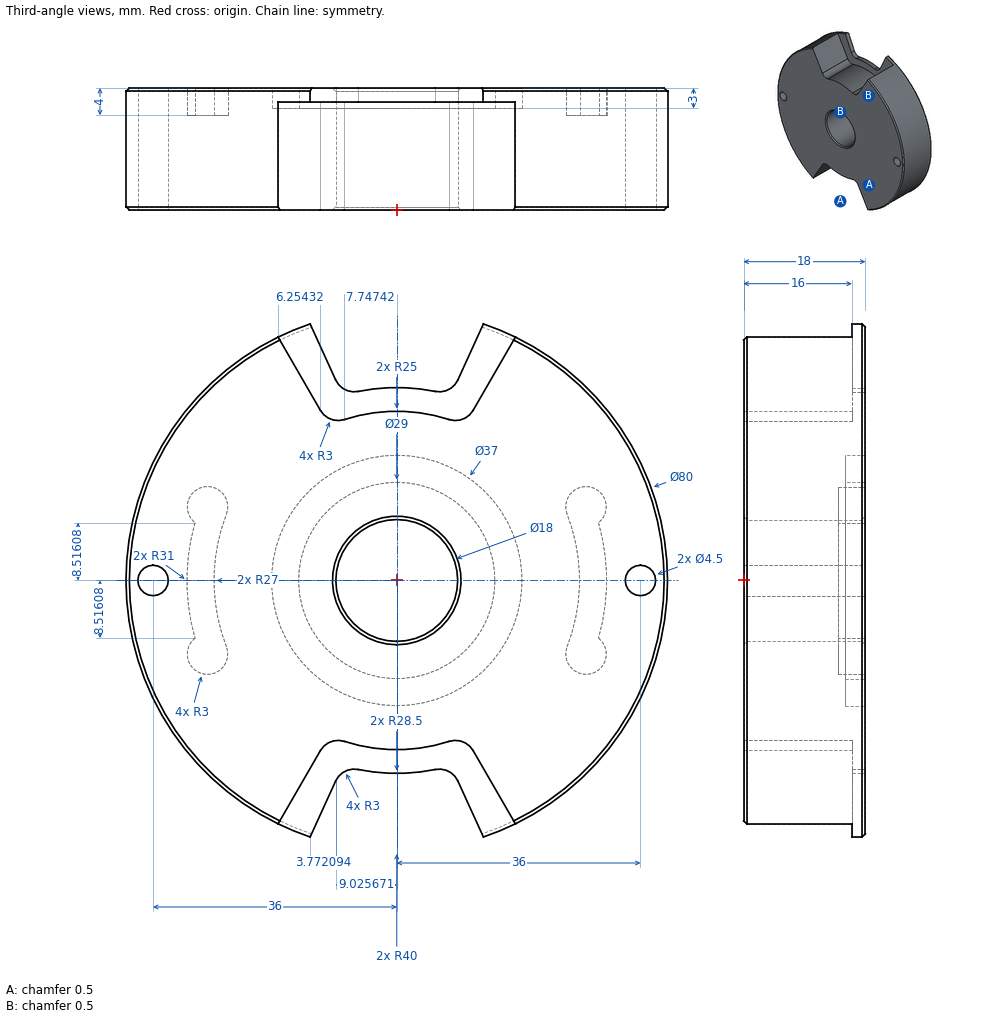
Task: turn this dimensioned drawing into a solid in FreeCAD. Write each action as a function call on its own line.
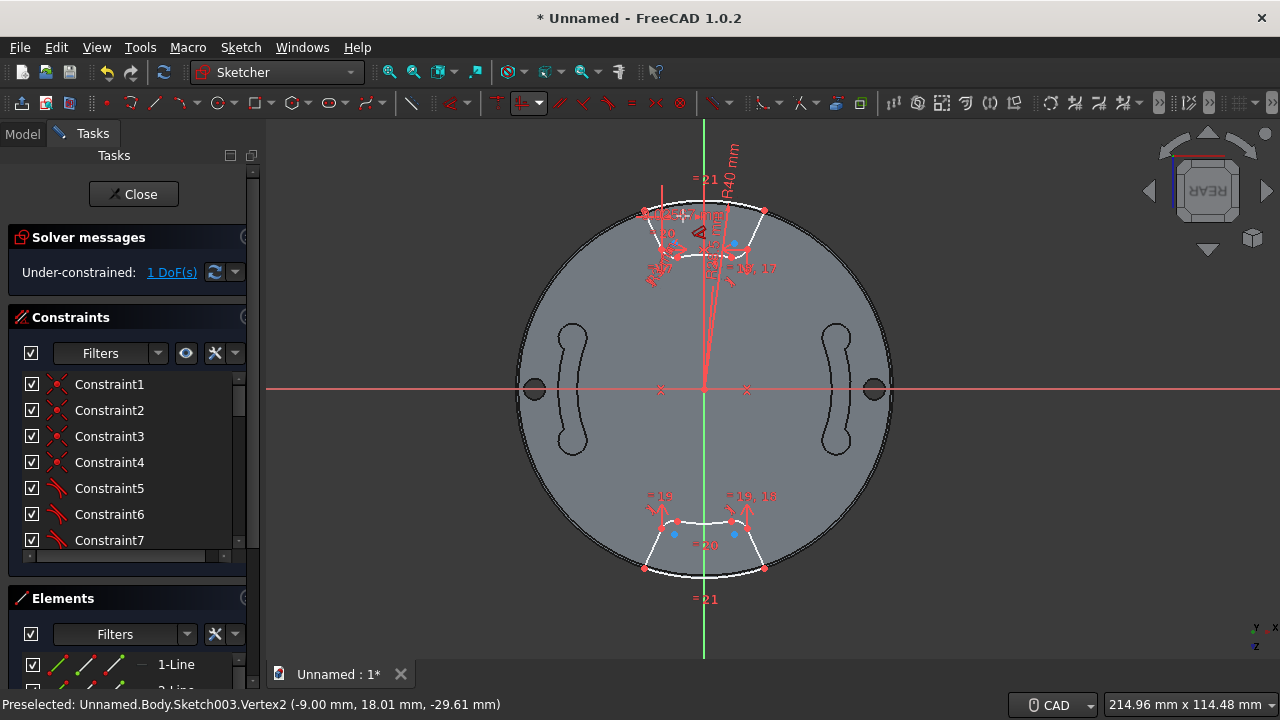
scroll(649, 222, up, 5)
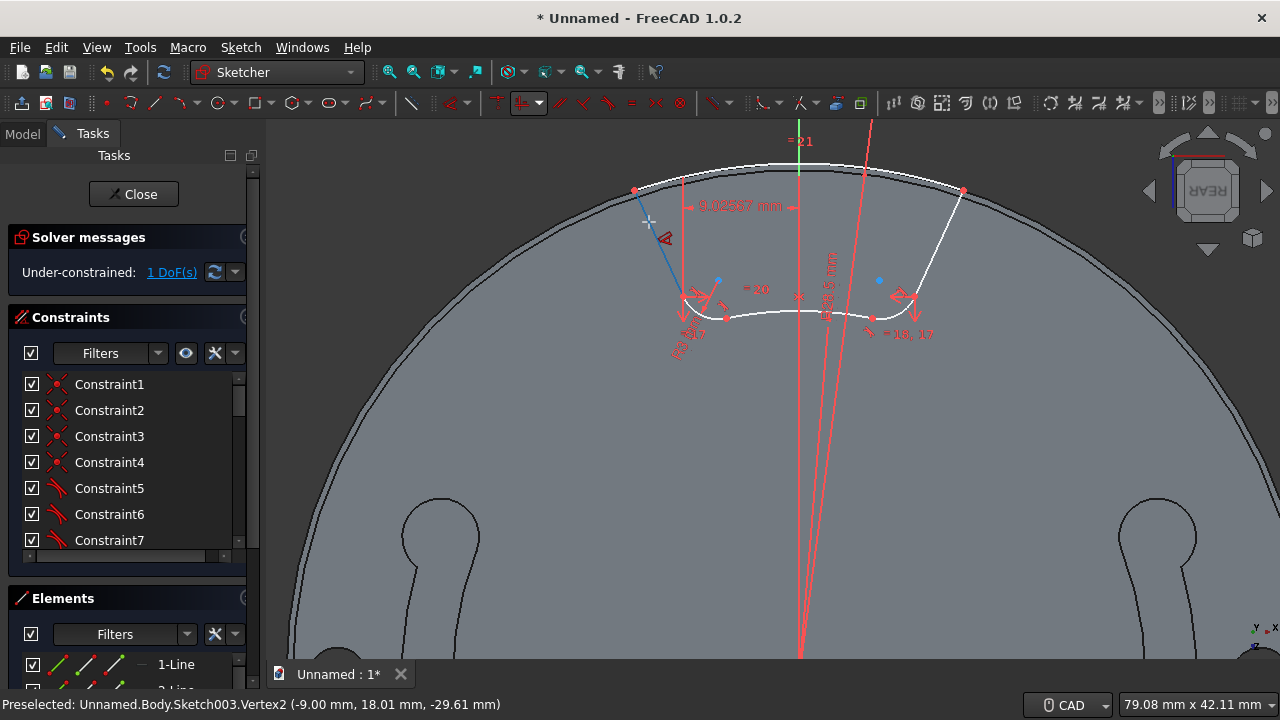
click(649, 222)
click(659, 157)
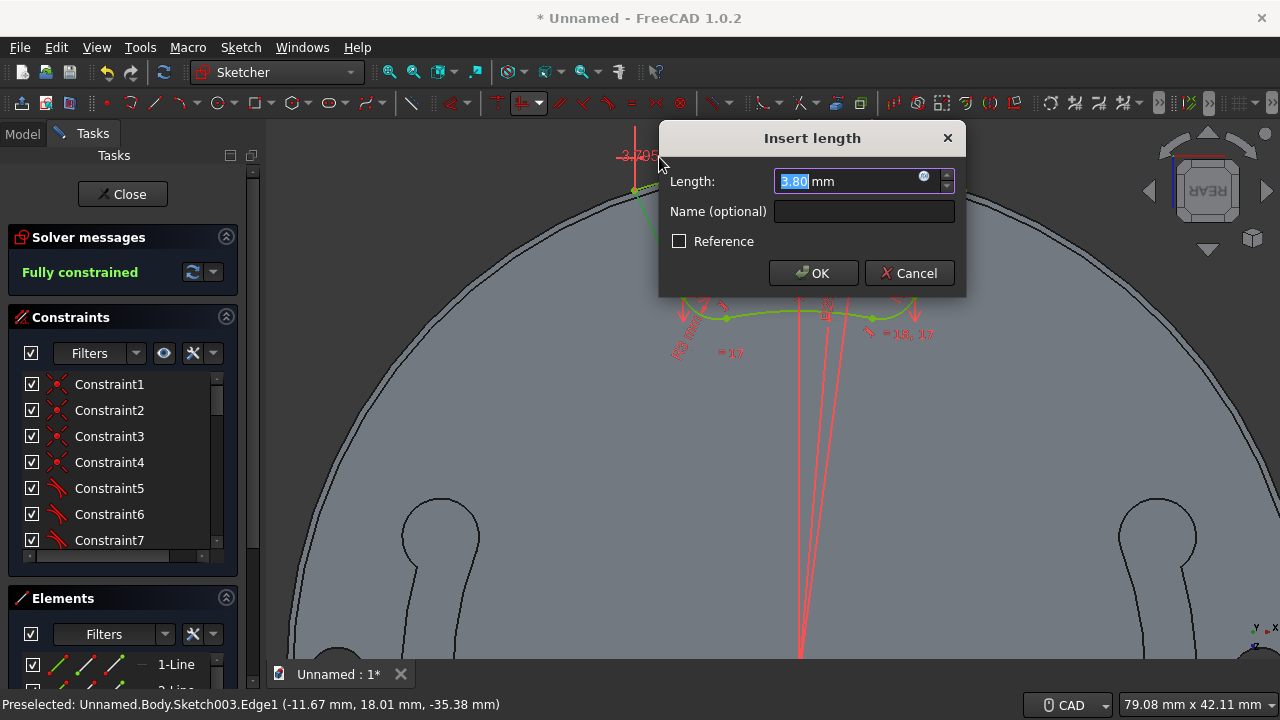
text(3.772094)
key(Return)
key(Escape)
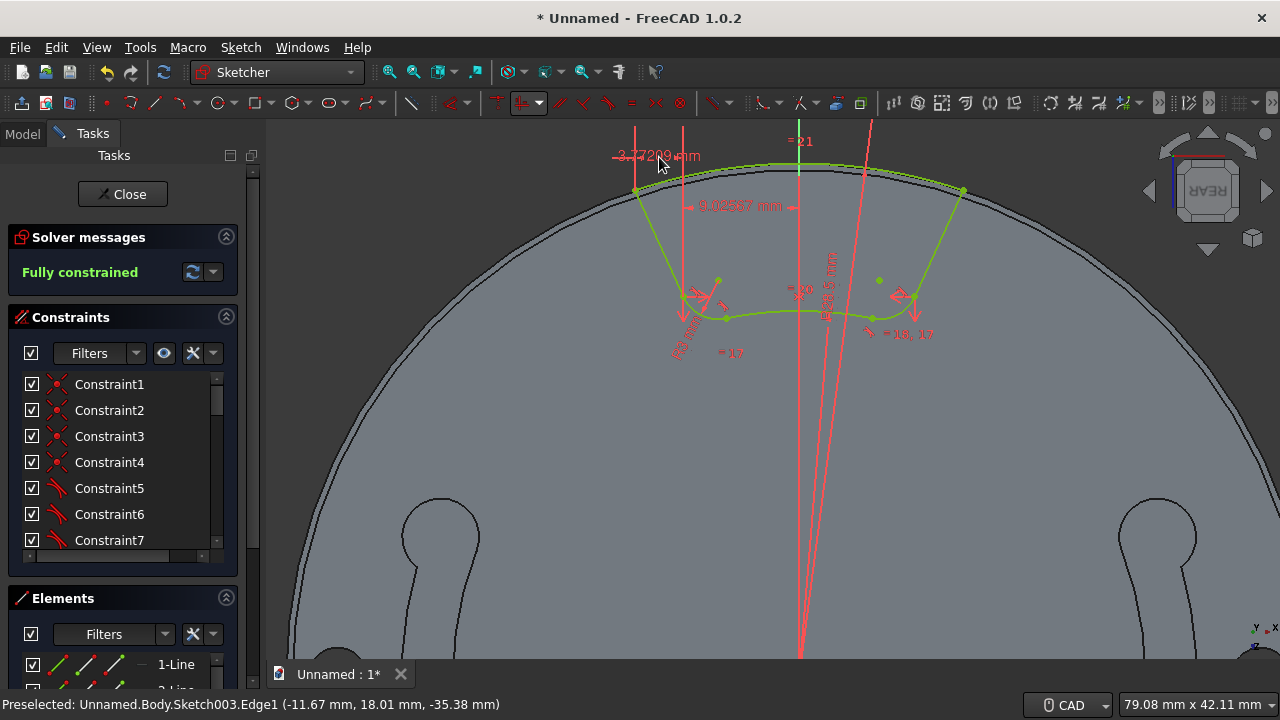
click(123, 194)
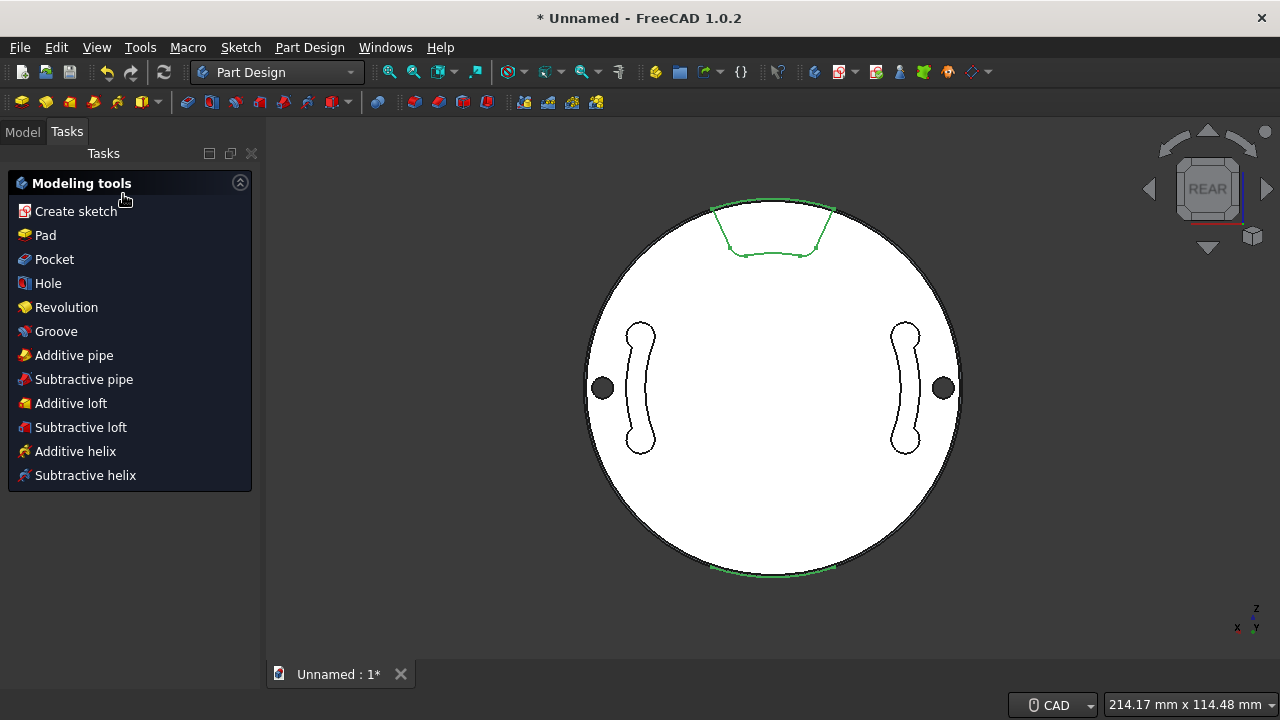
click(188, 102)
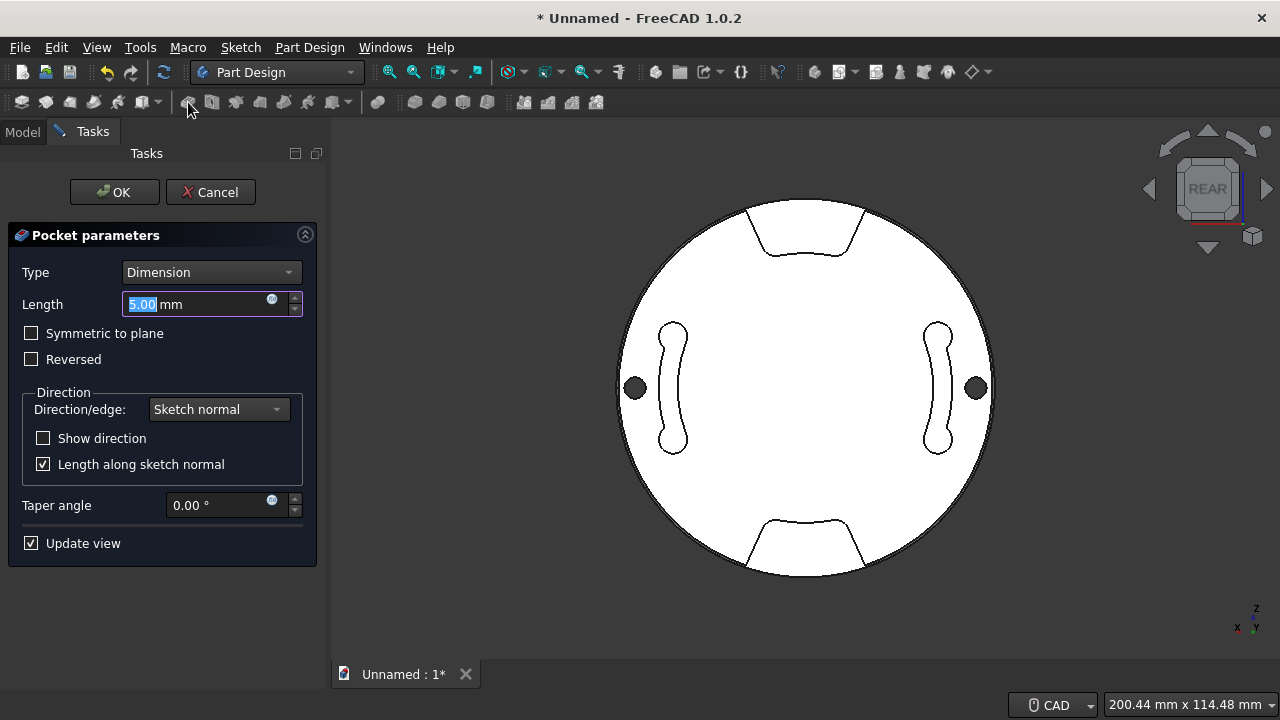
click(212, 272)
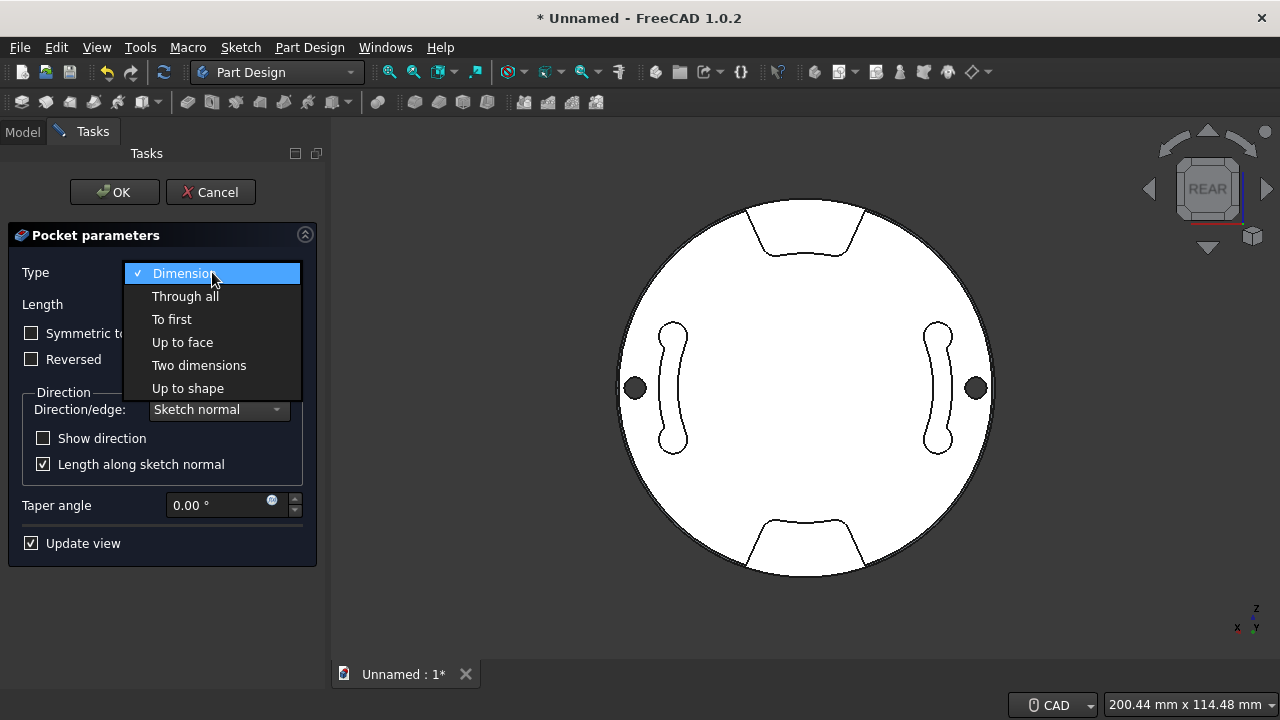
click(212, 296)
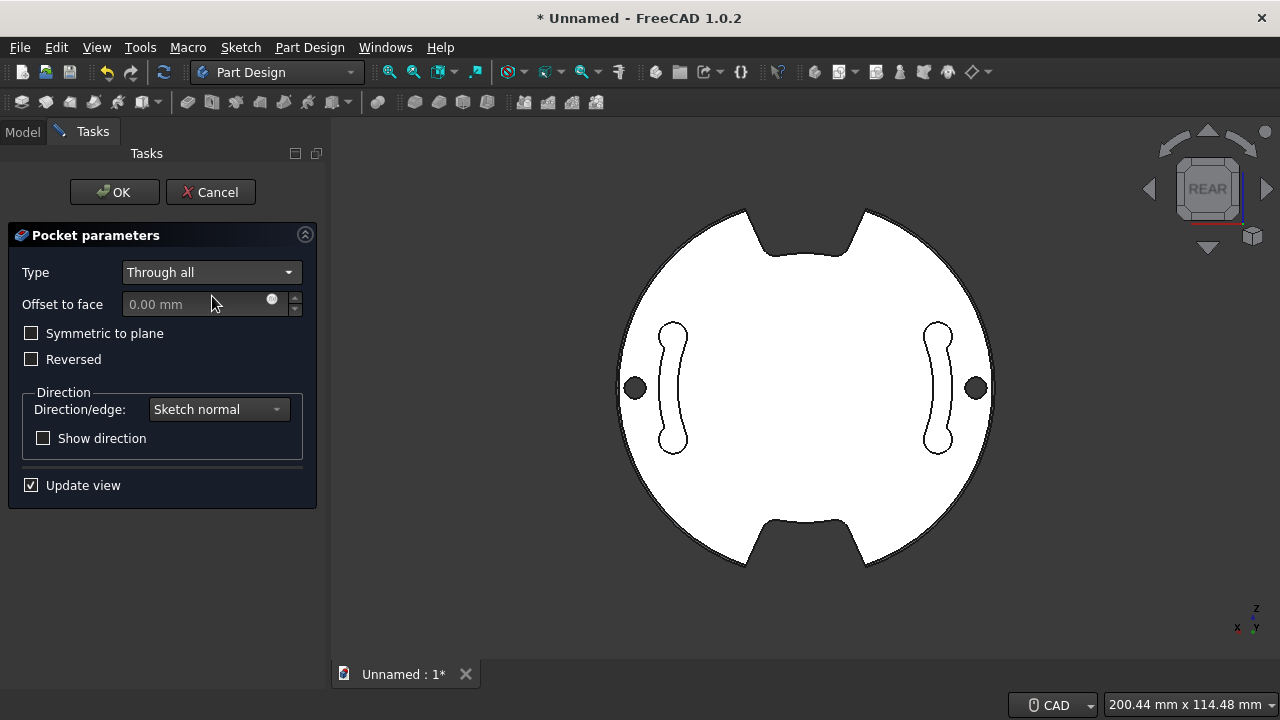
click(115, 192)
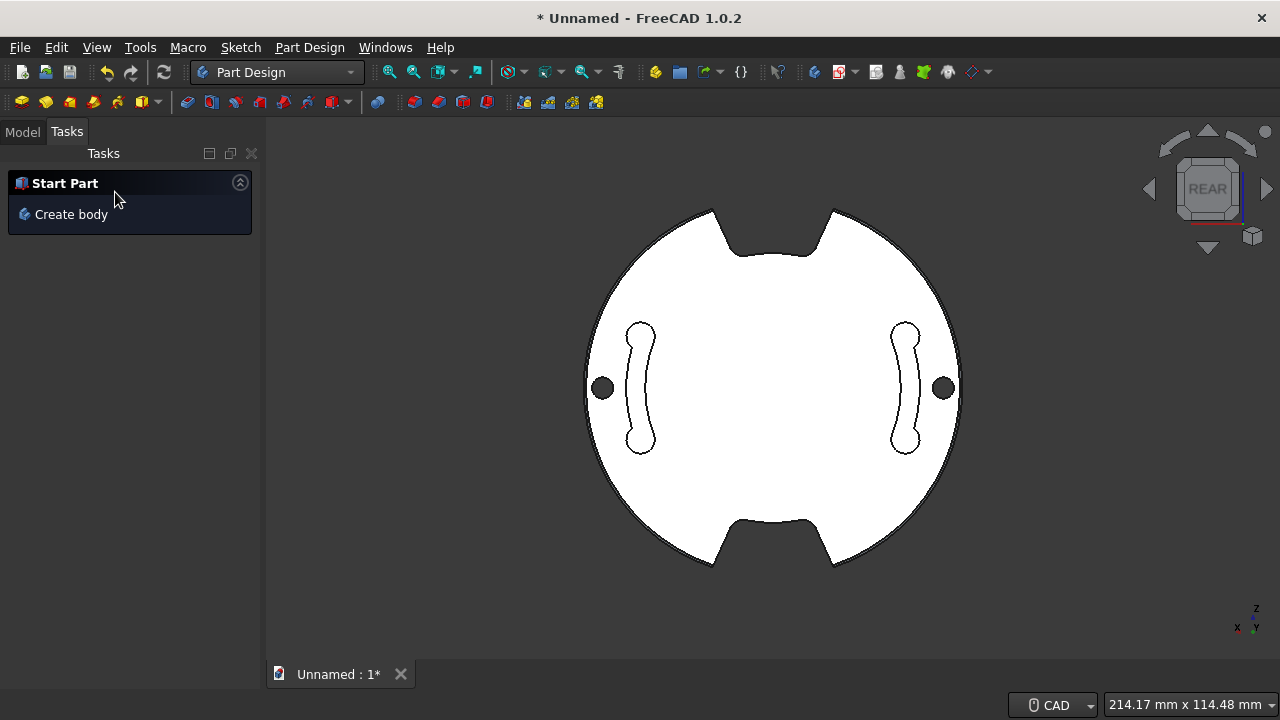
click(840, 72)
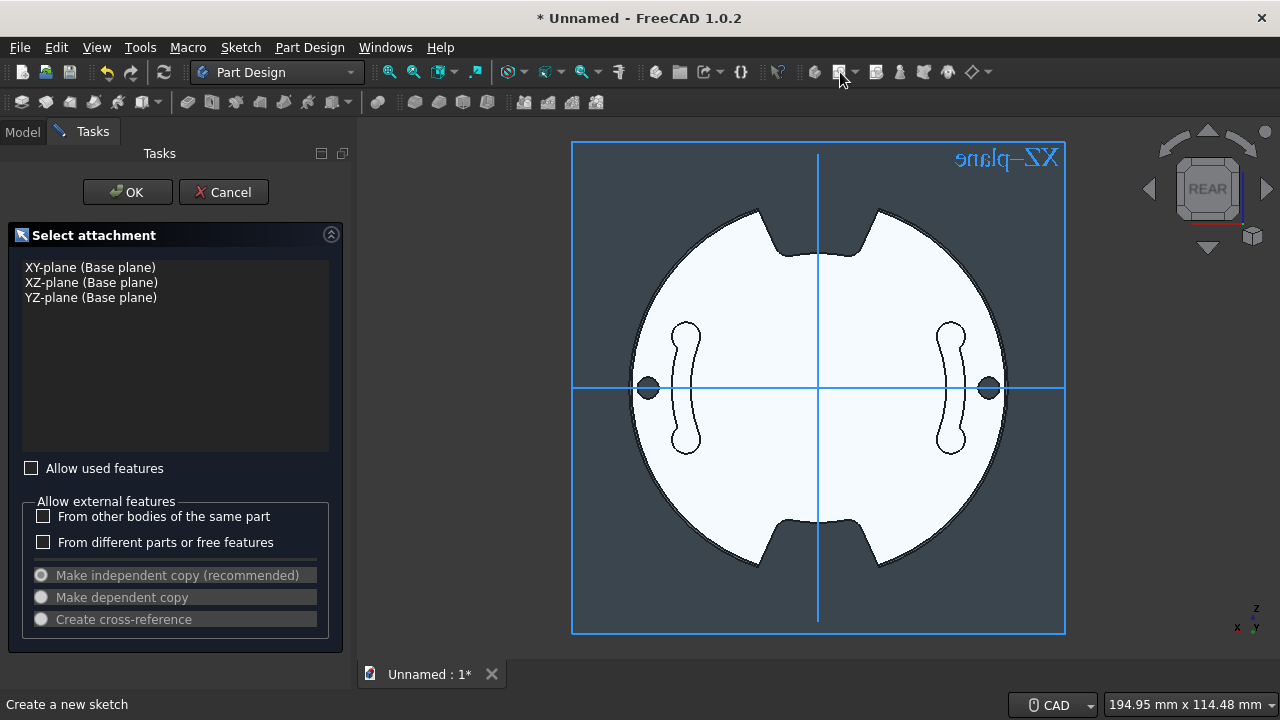
click(82, 282)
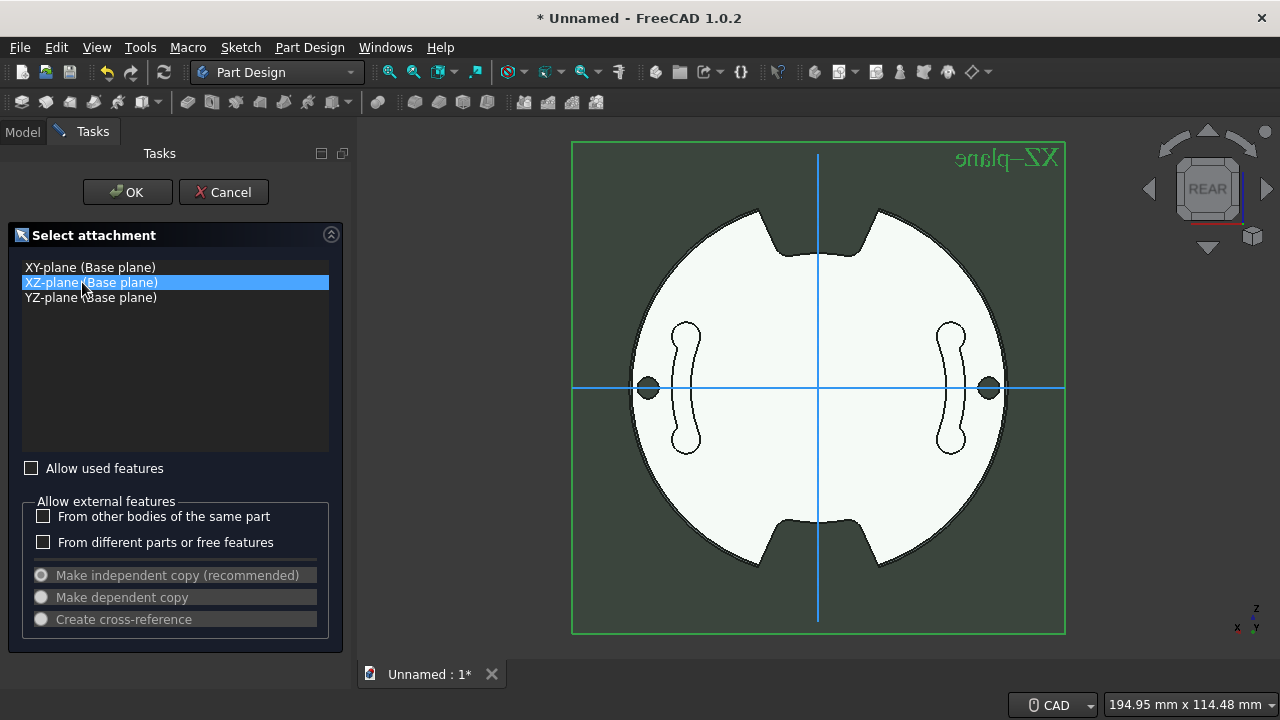
click(128, 192)